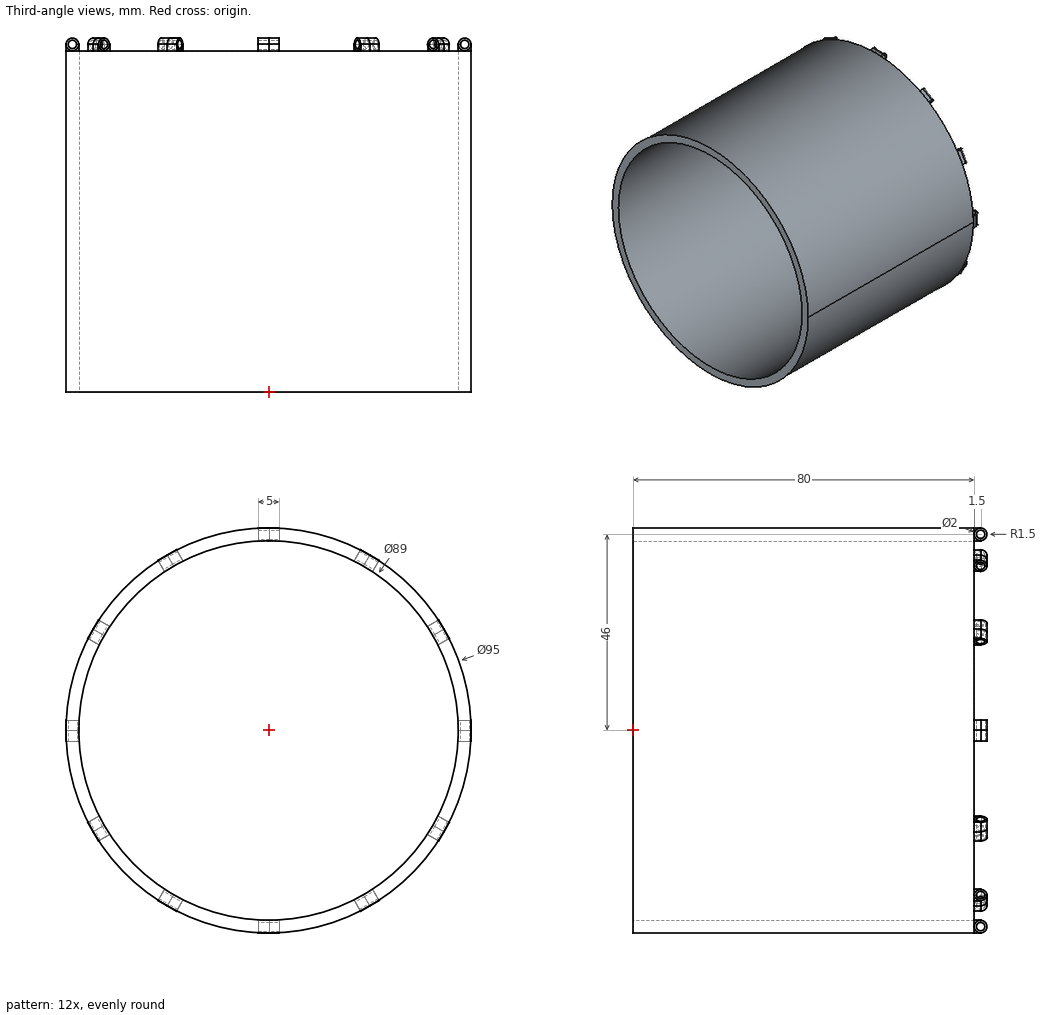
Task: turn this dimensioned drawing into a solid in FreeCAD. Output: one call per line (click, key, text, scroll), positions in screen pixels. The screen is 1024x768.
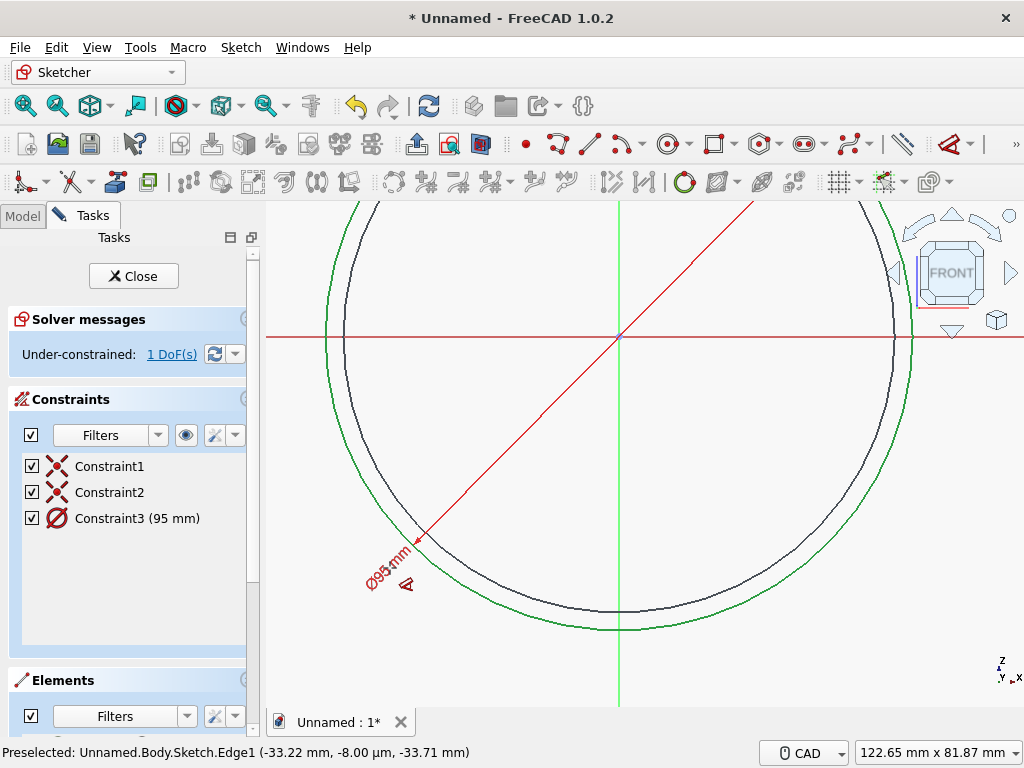
click(425, 532)
click(325, 424)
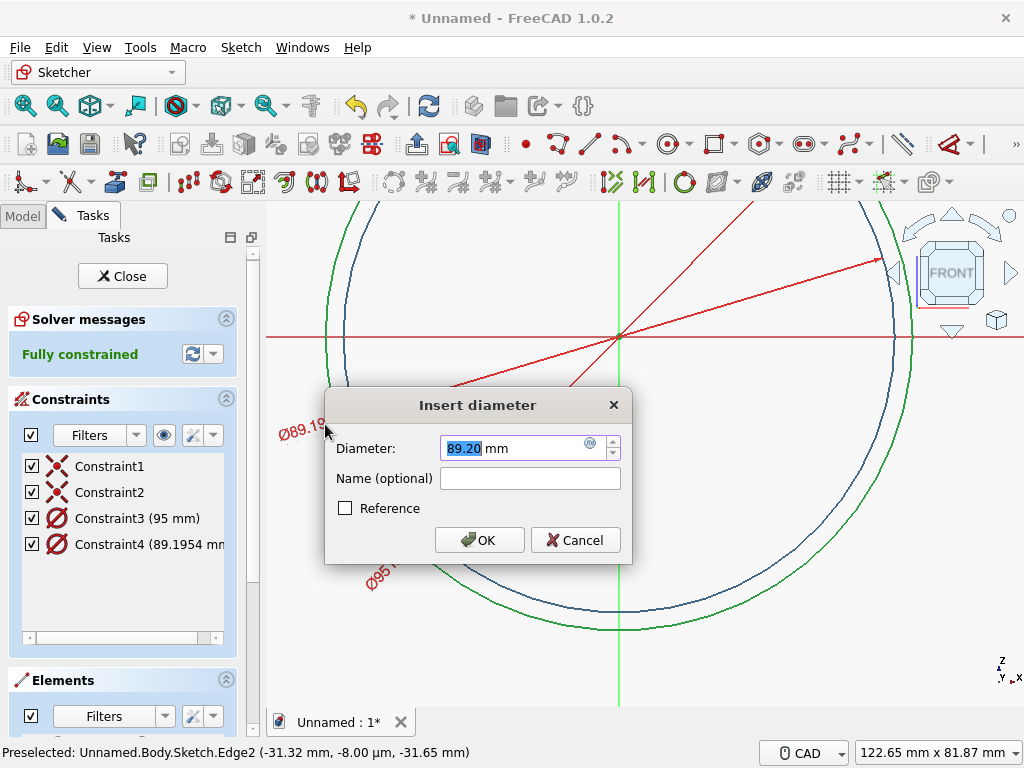
text(89)
key(Return)
key(Escape)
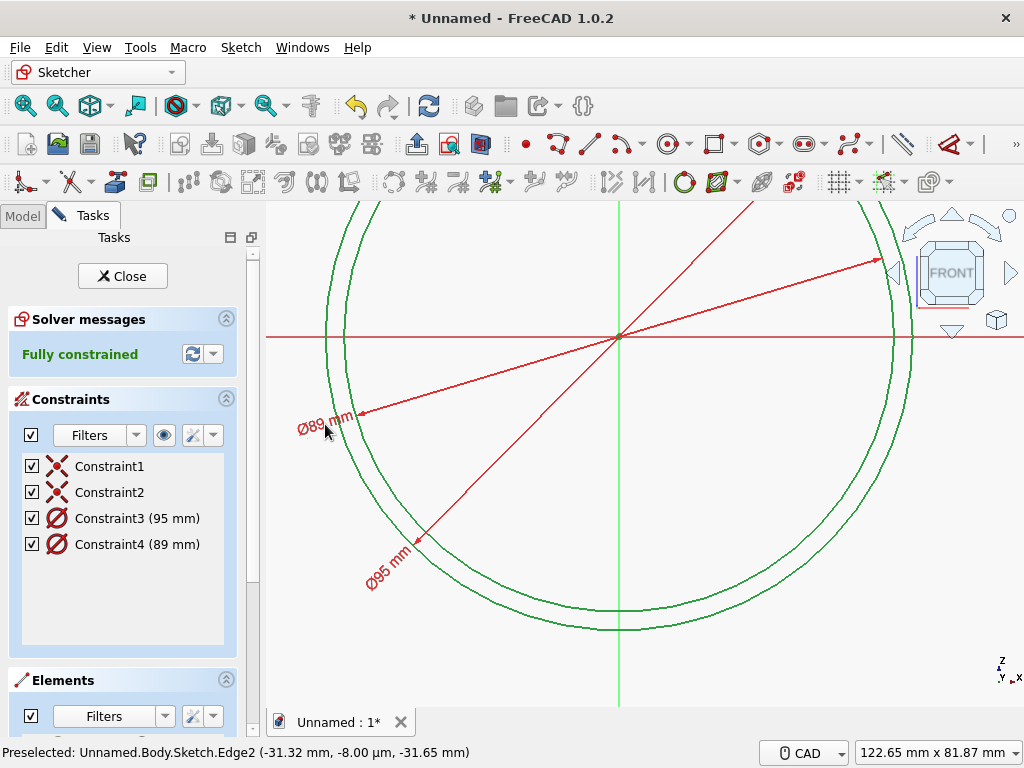
click(123, 276)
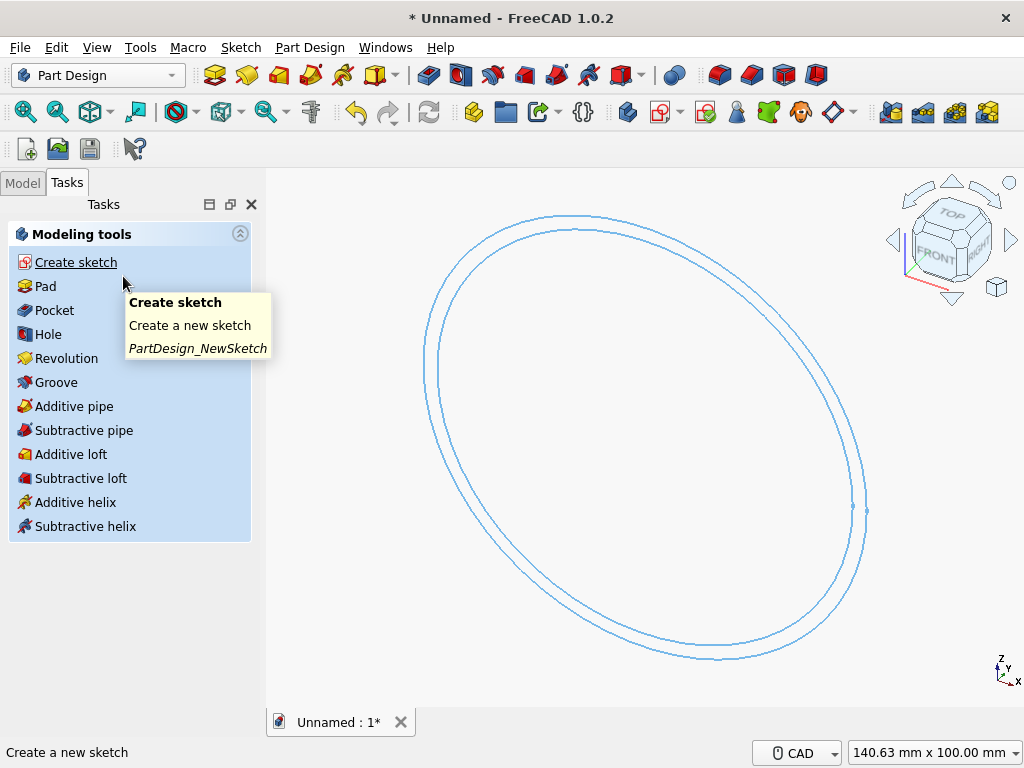
click(216, 76)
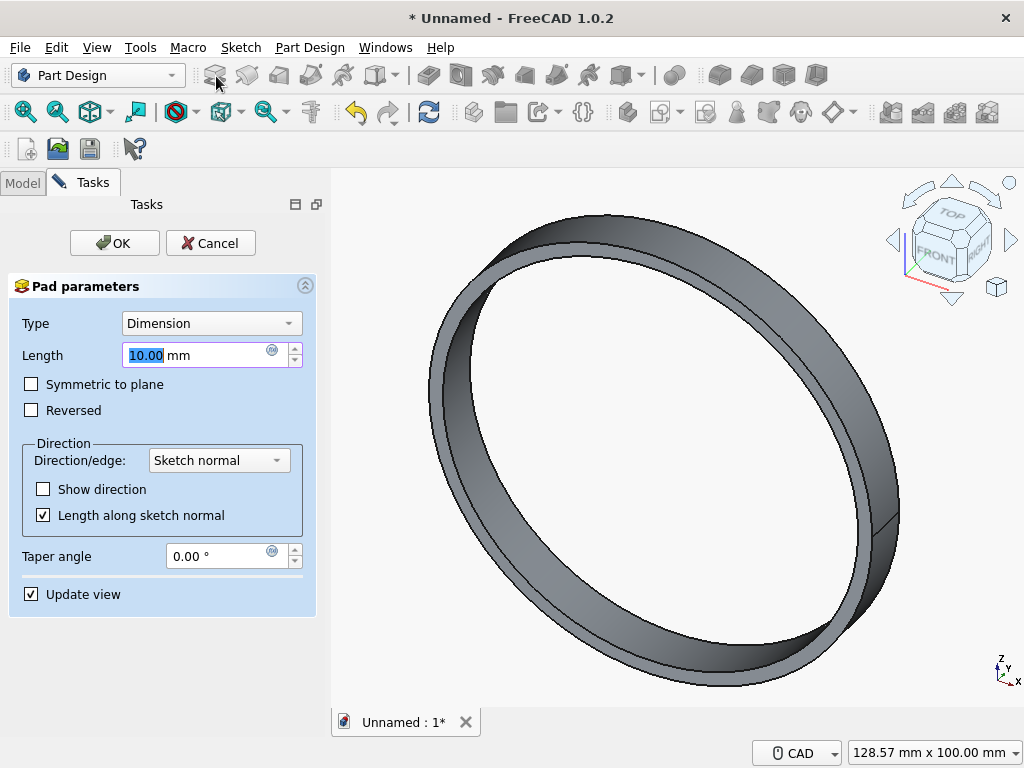
text(80)
key(Tab)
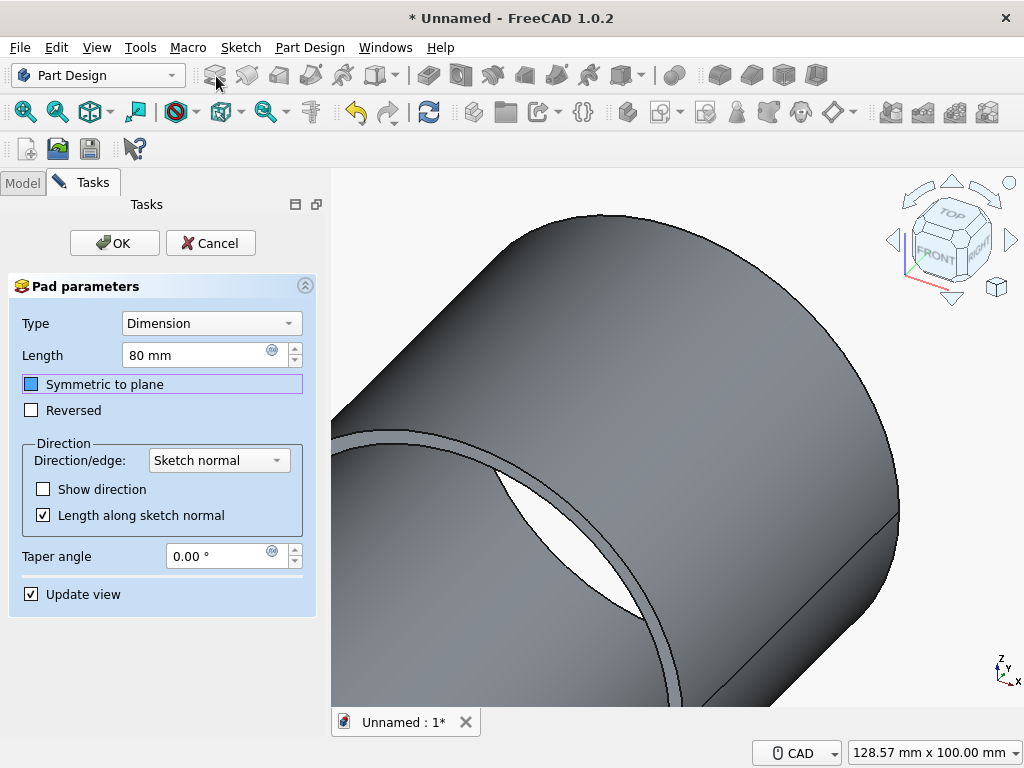
click(30, 410)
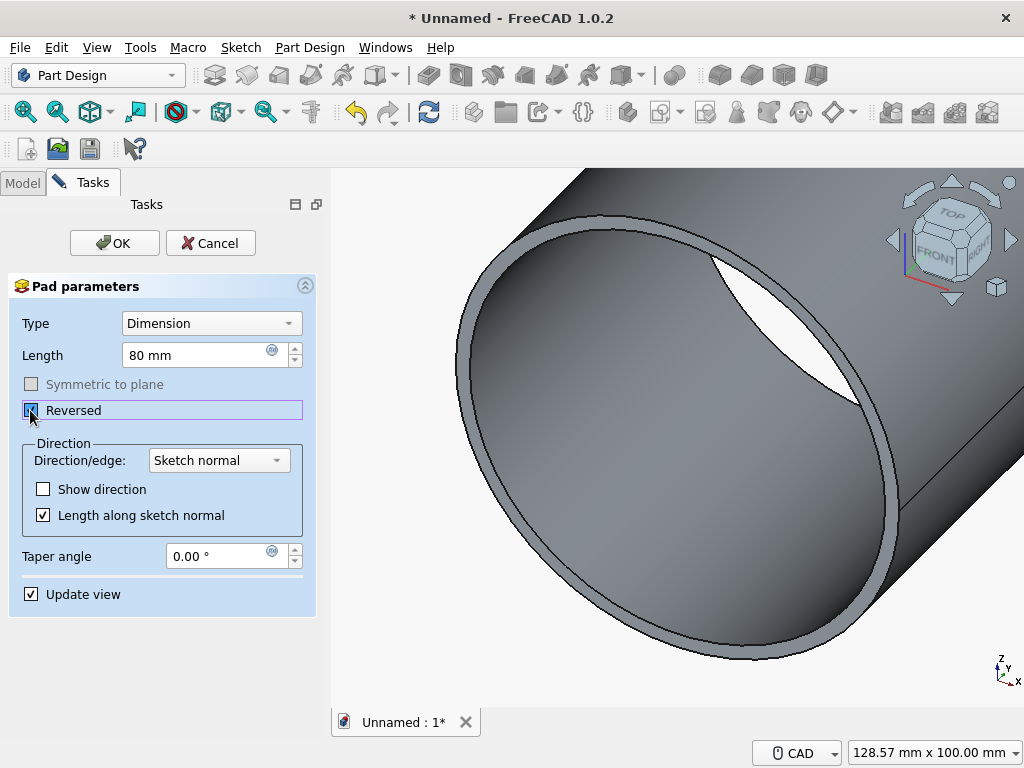
click(115, 243)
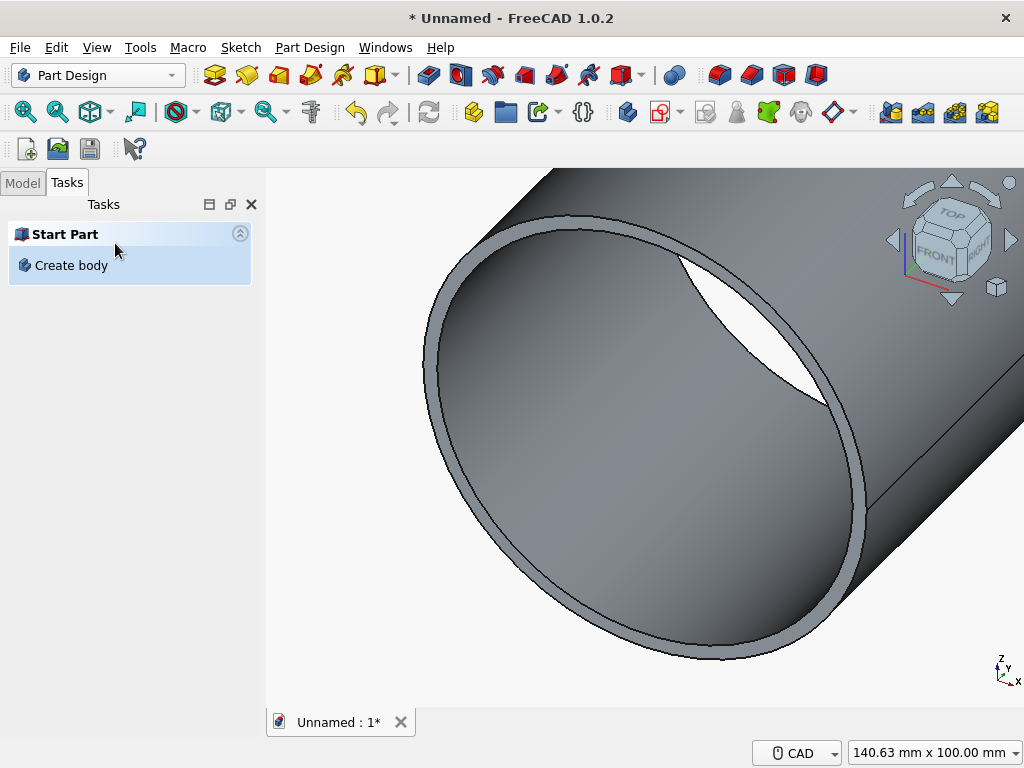
key(v)
key(f)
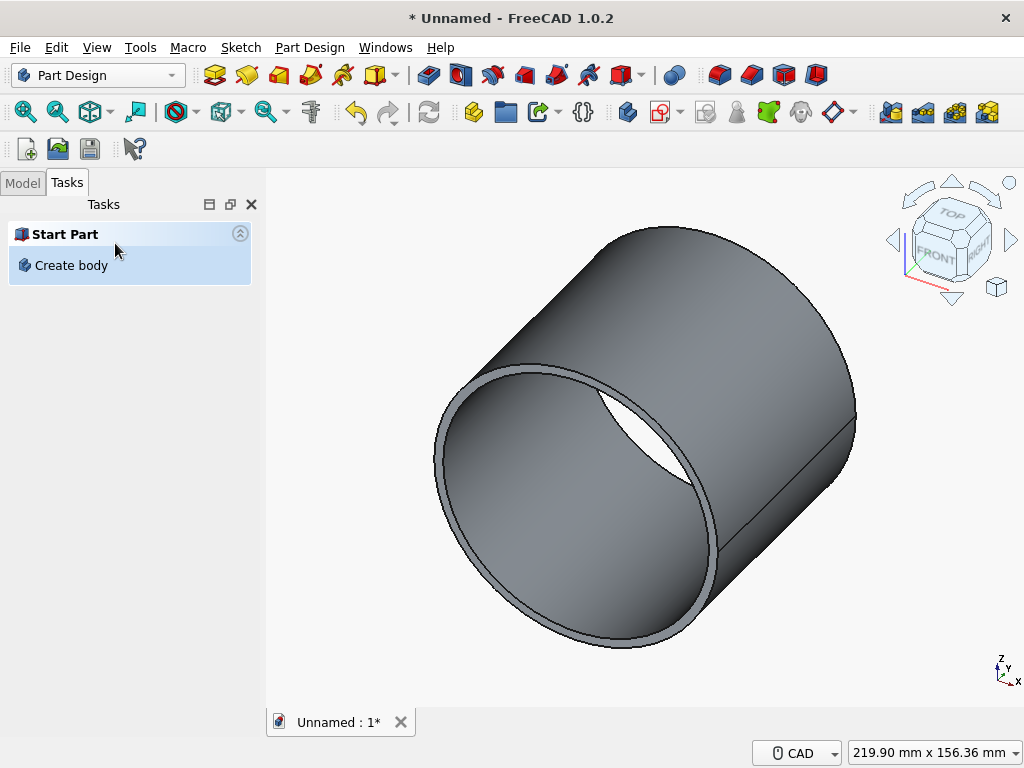
click(660, 112)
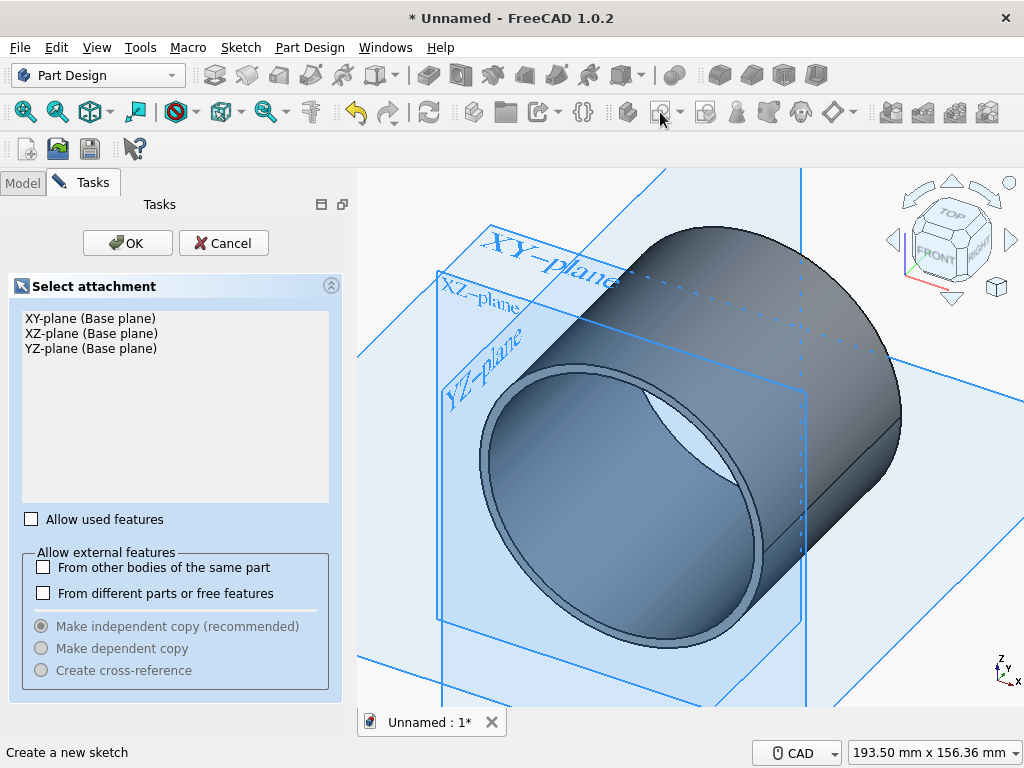
click(82, 348)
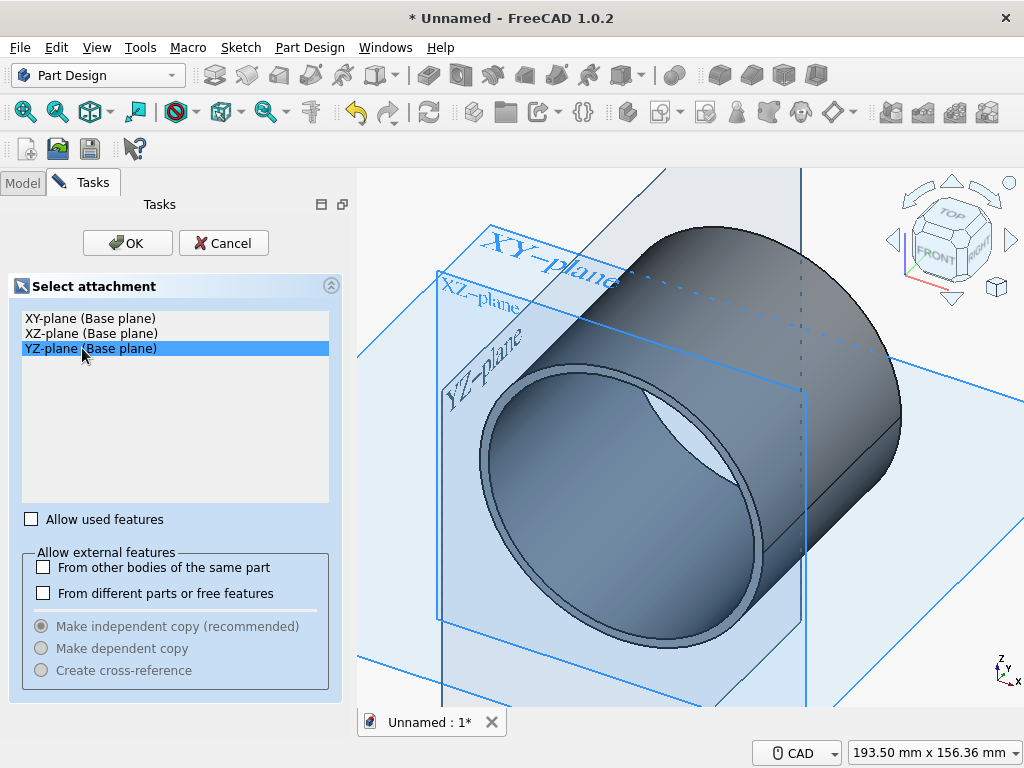
click(128, 243)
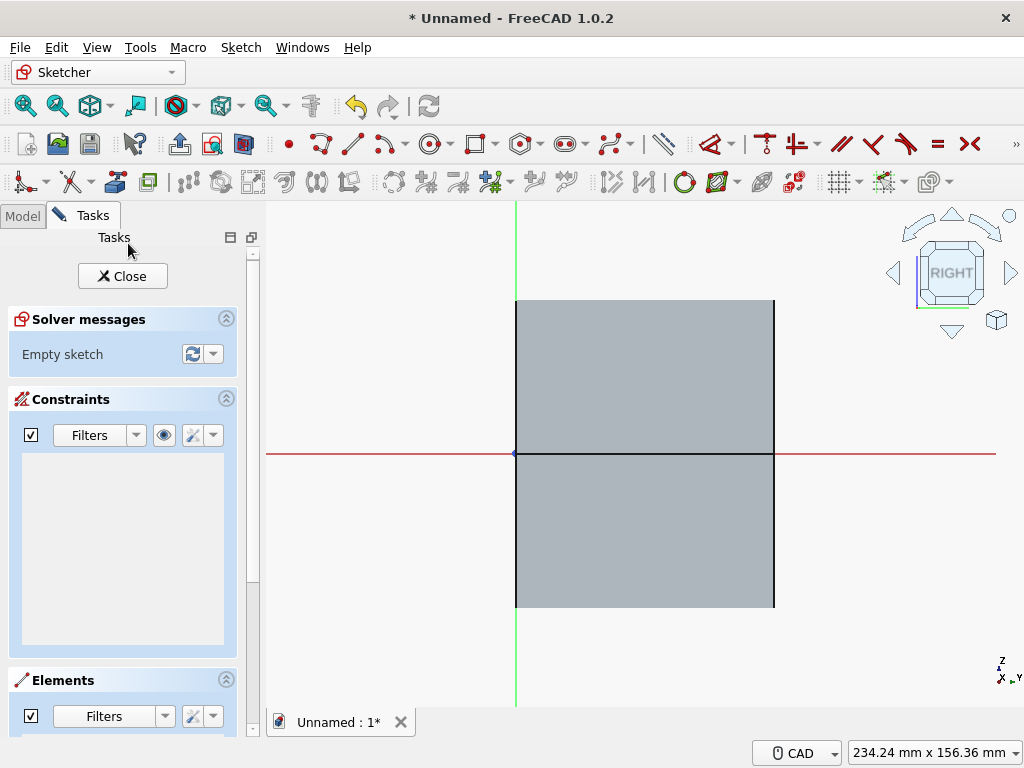
click(244, 144)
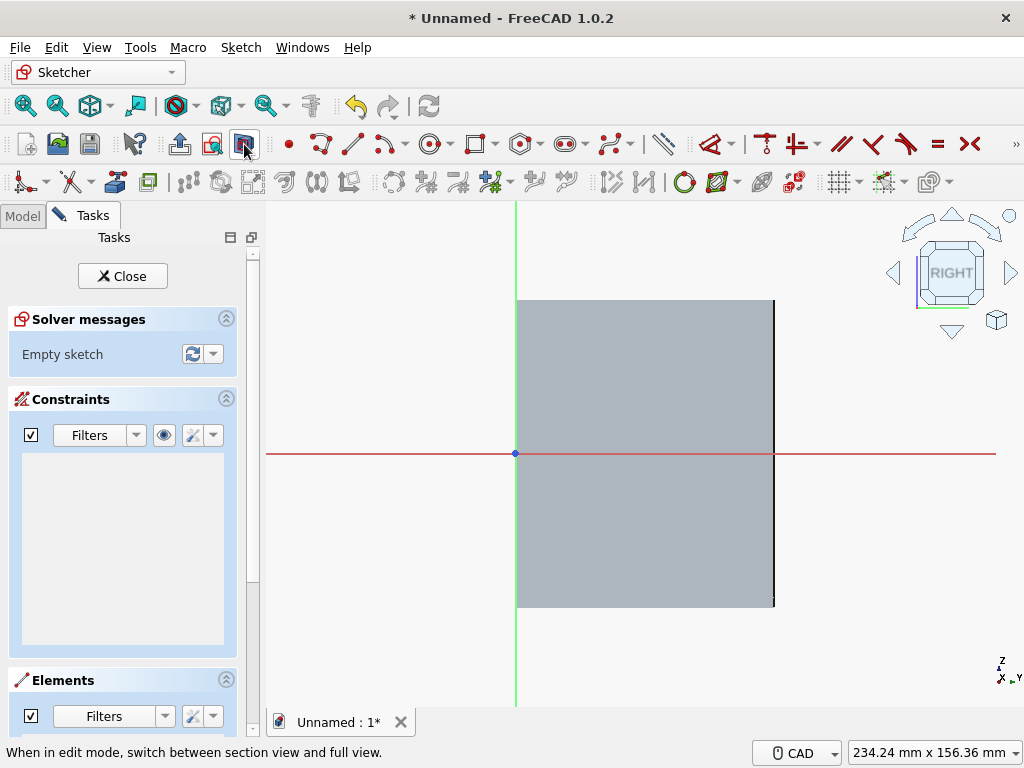
scroll(790, 297, up, 15)